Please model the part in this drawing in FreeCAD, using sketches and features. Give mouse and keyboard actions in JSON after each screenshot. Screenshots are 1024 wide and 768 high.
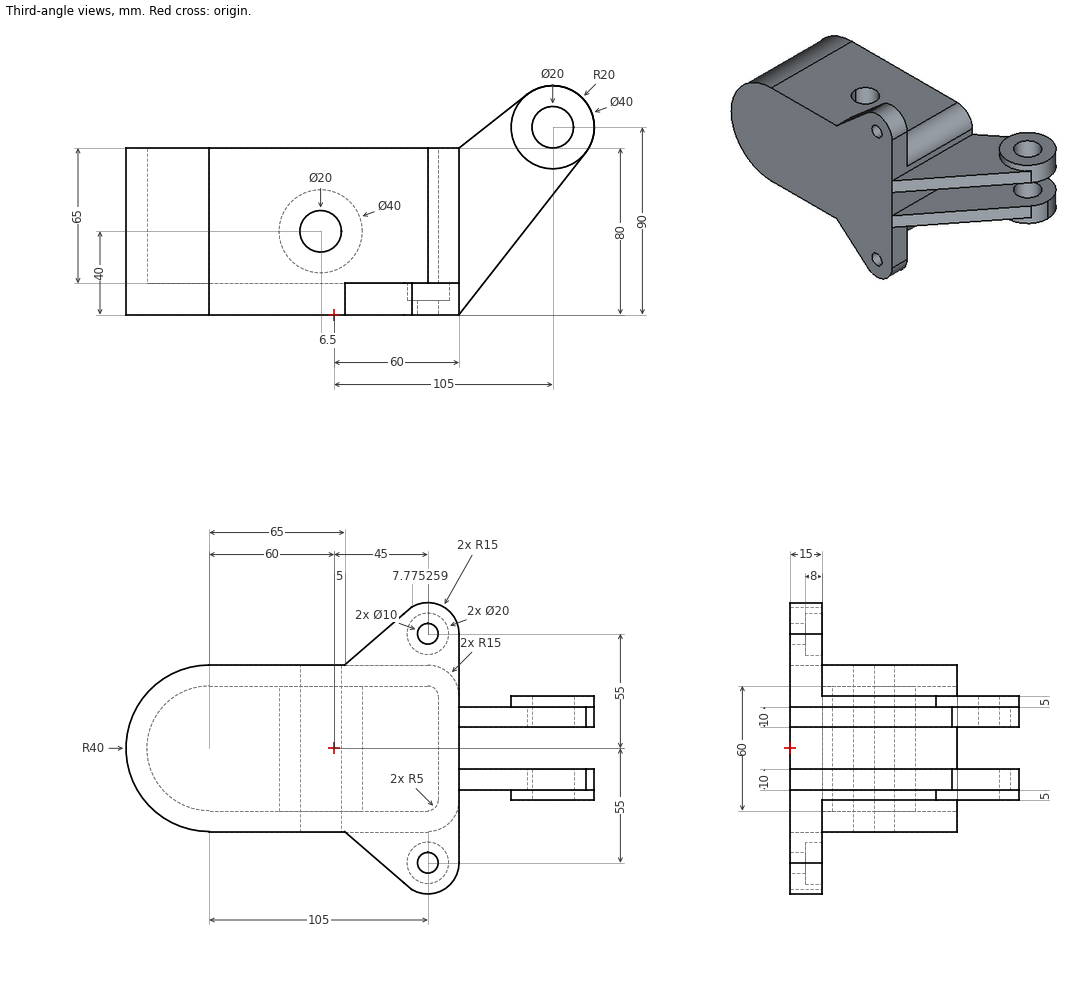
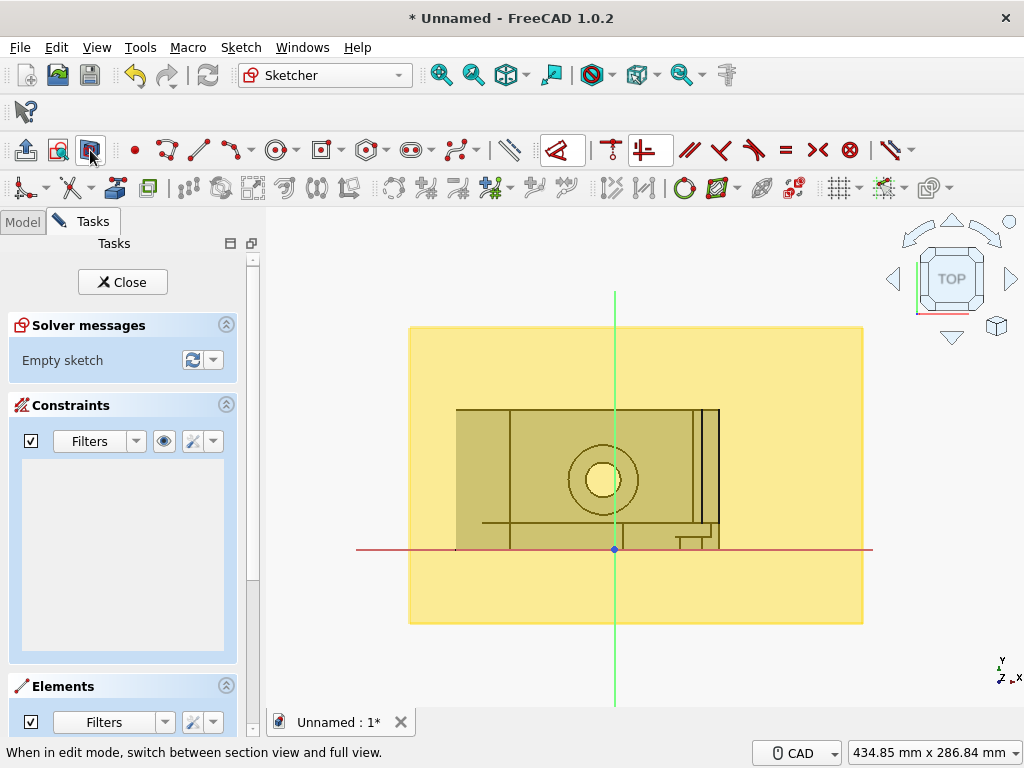
{"action": "scroll", "coordinate": [854, 376], "scroll_direction": "up", "scroll_amount": 8}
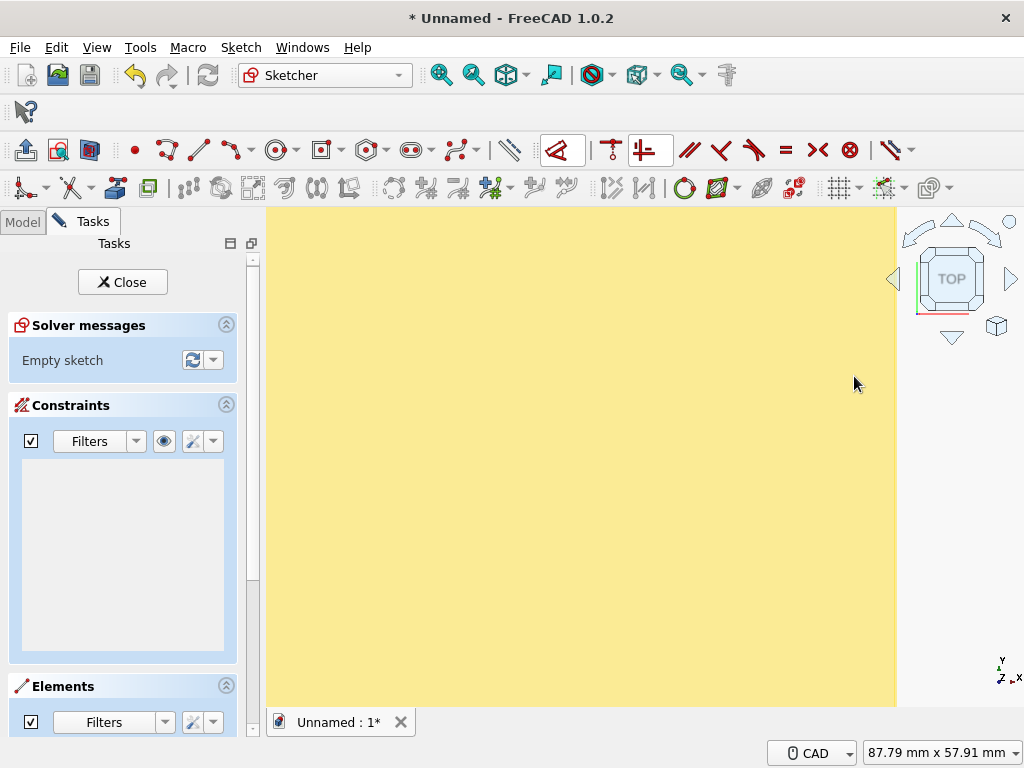
{"action": "left_click", "coordinate": [276, 150]}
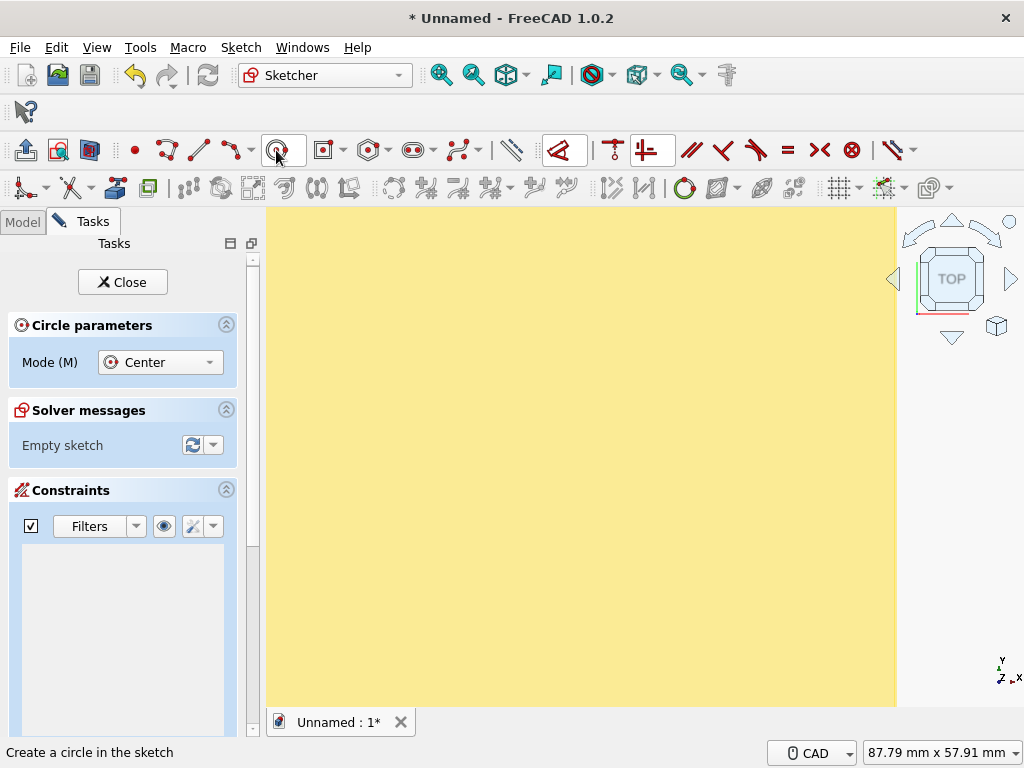
{"action": "left_click", "coordinate": [572, 458]}
{"action": "left_click", "coordinate": [694, 335]}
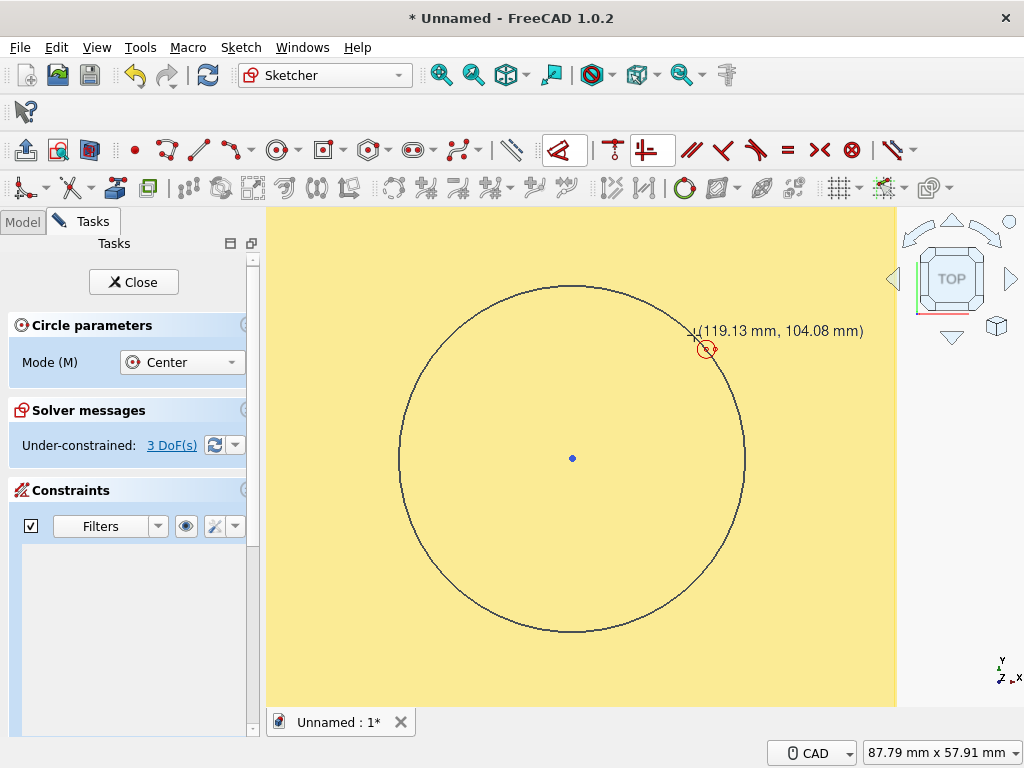
{"action": "left_click", "coordinate": [572, 459]}
{"action": "left_click", "coordinate": [633, 397]}
{"action": "key", "text": "Escape"}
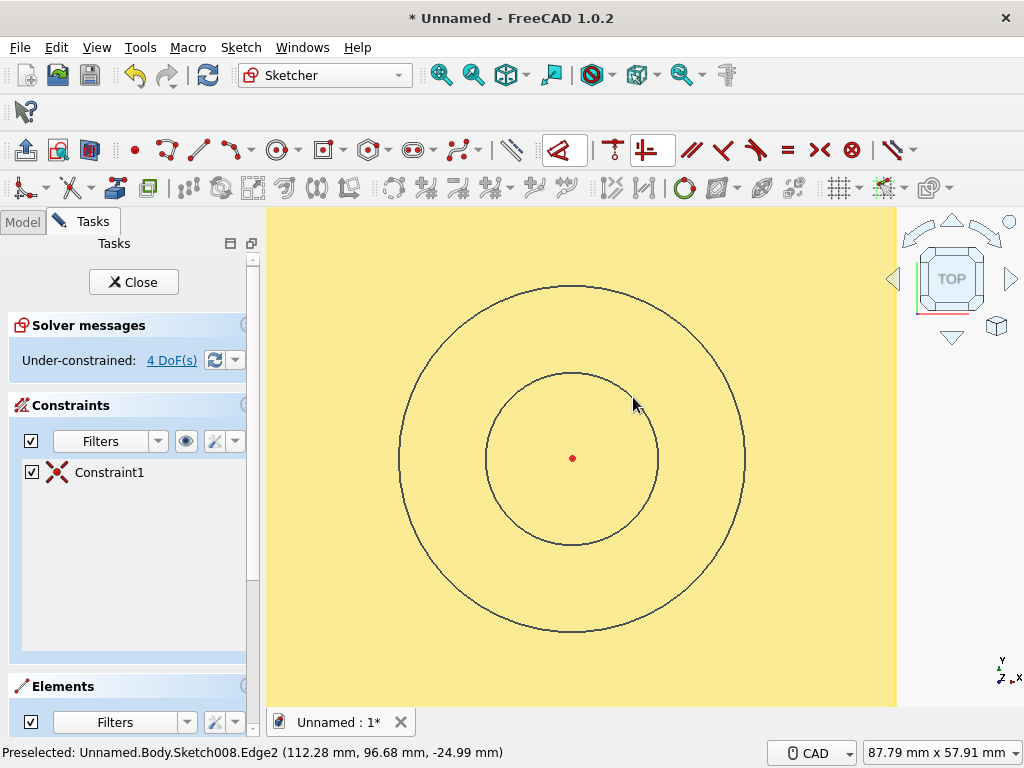
{"action": "left_click", "coordinate": [694, 336]}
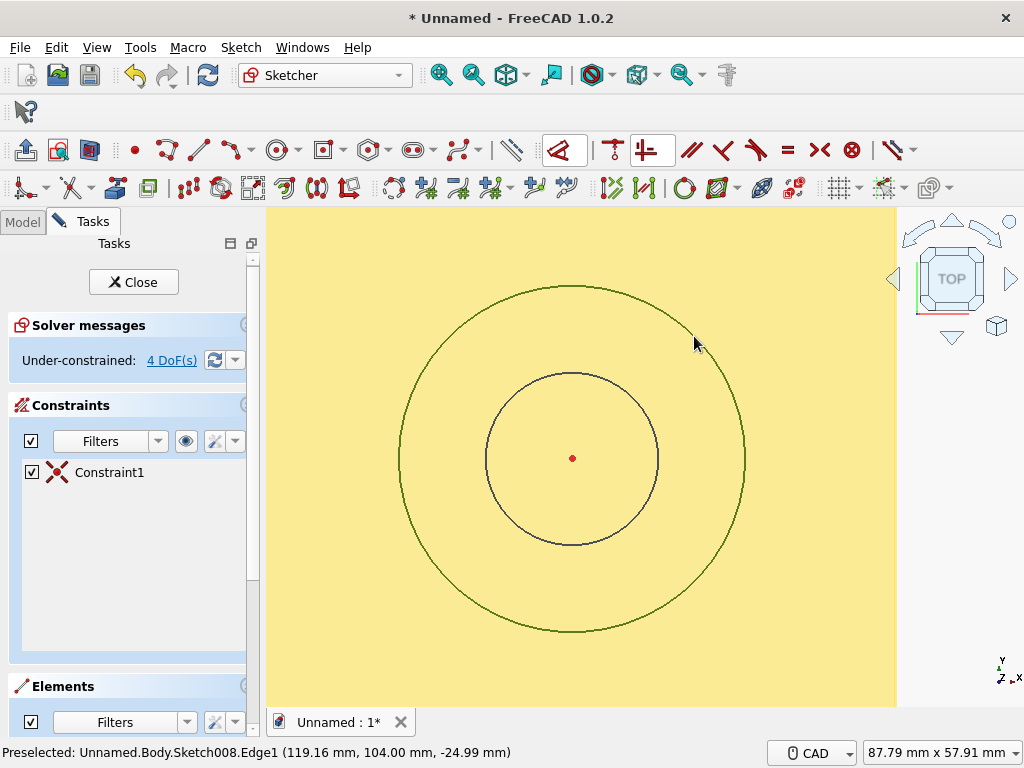
{"action": "key", "text": "k o"}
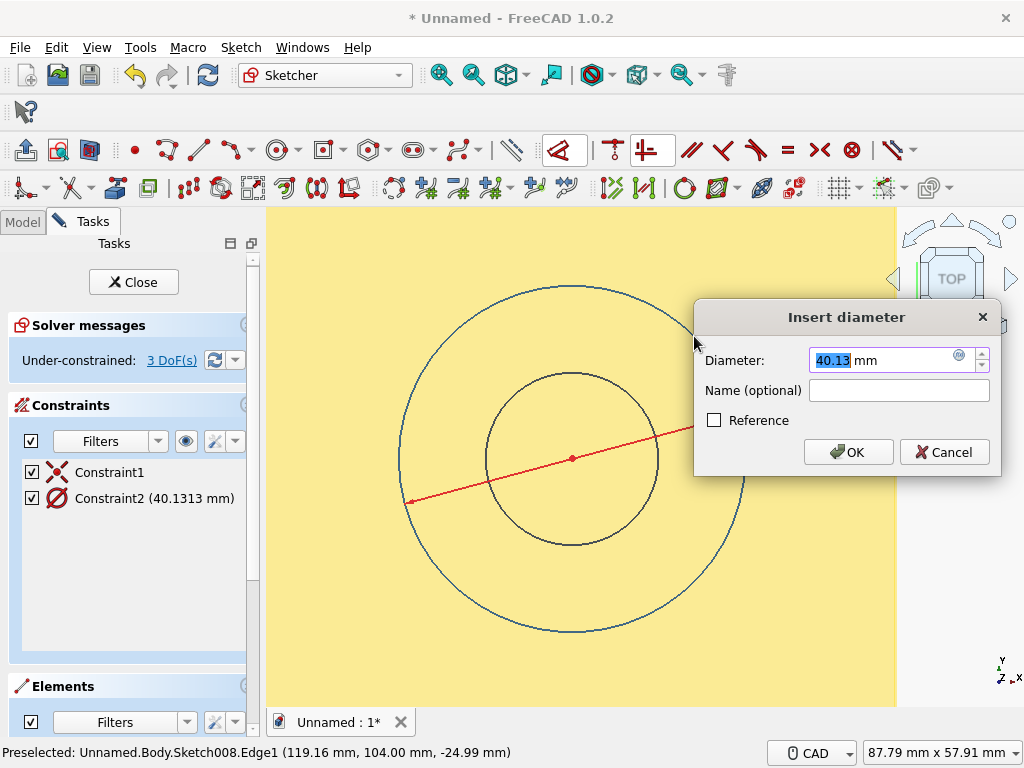
{"action": "type", "text": "40"}
{"action": "key", "text": "Return"}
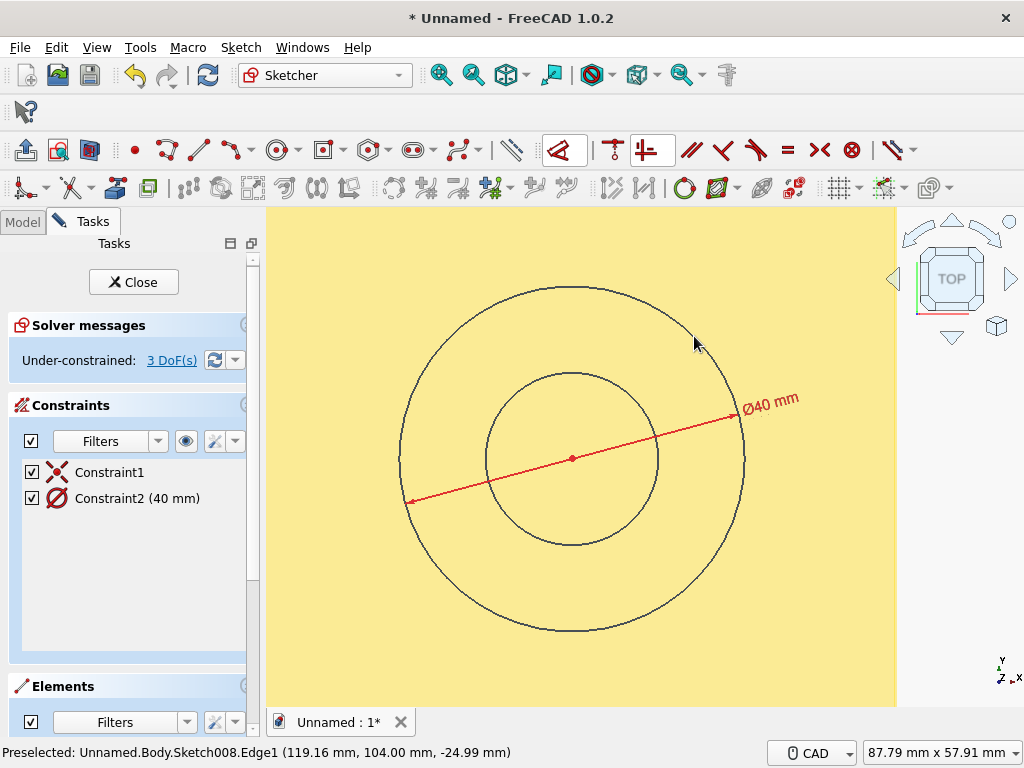
{"action": "left_click", "coordinate": [633, 398]}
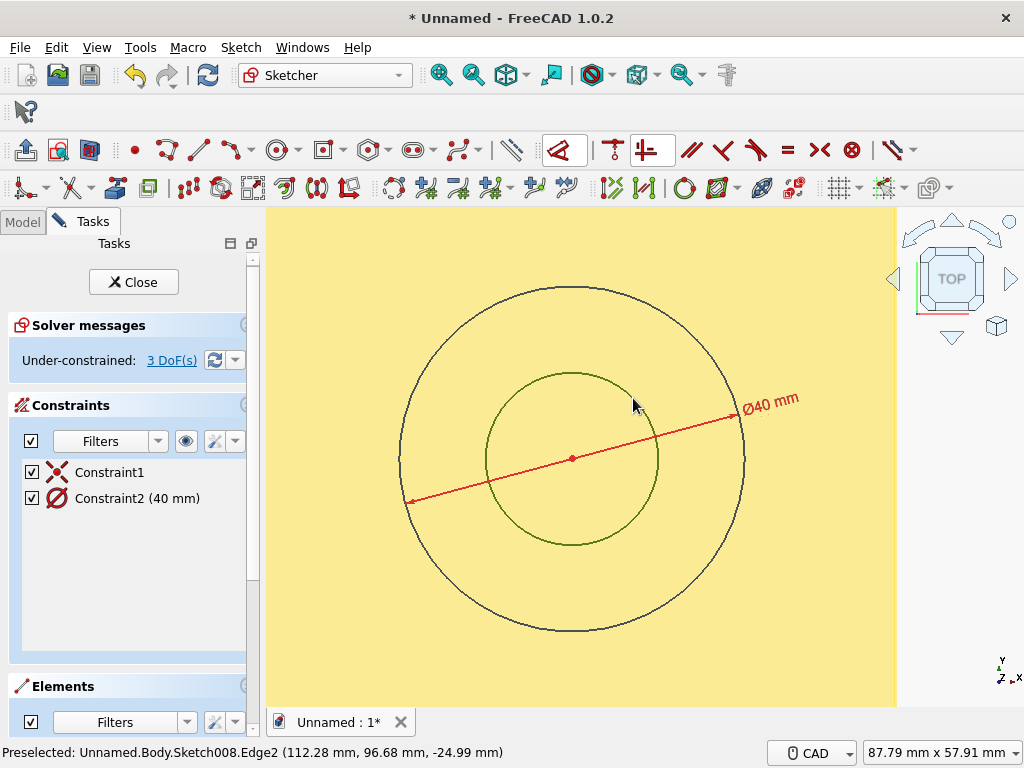
{"action": "key", "text": "k o"}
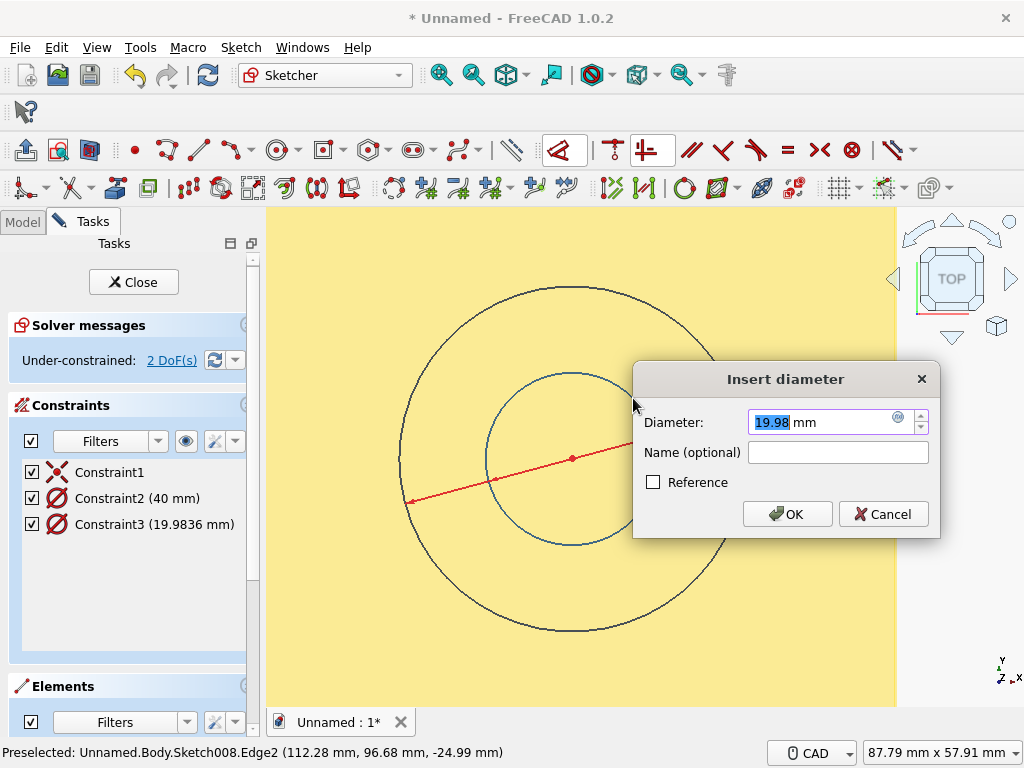
{"action": "type", "text": "20"}
{"action": "key", "text": "Return"}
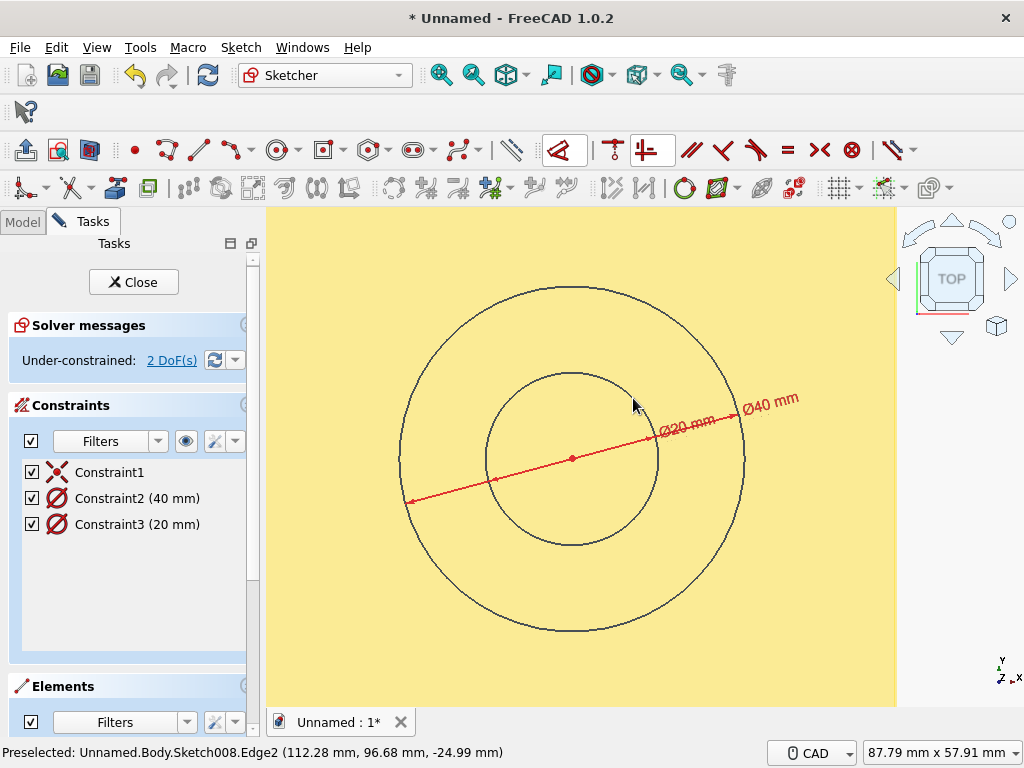
{"action": "left_click", "coordinate": [572, 459]}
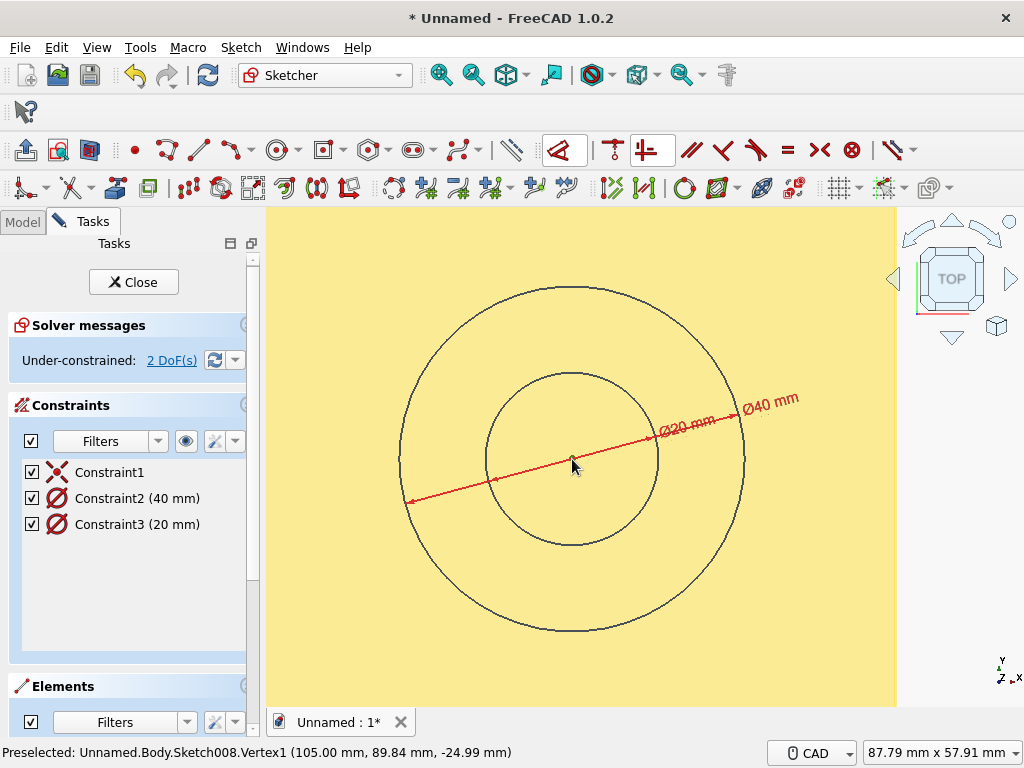
{"action": "left_click", "coordinate": [582, 150]}